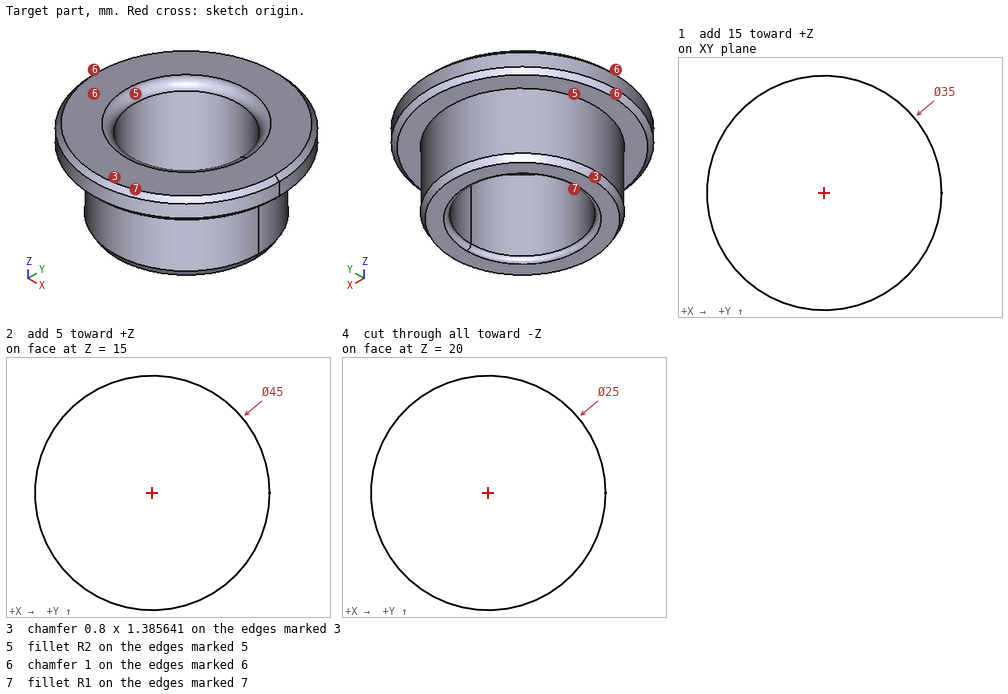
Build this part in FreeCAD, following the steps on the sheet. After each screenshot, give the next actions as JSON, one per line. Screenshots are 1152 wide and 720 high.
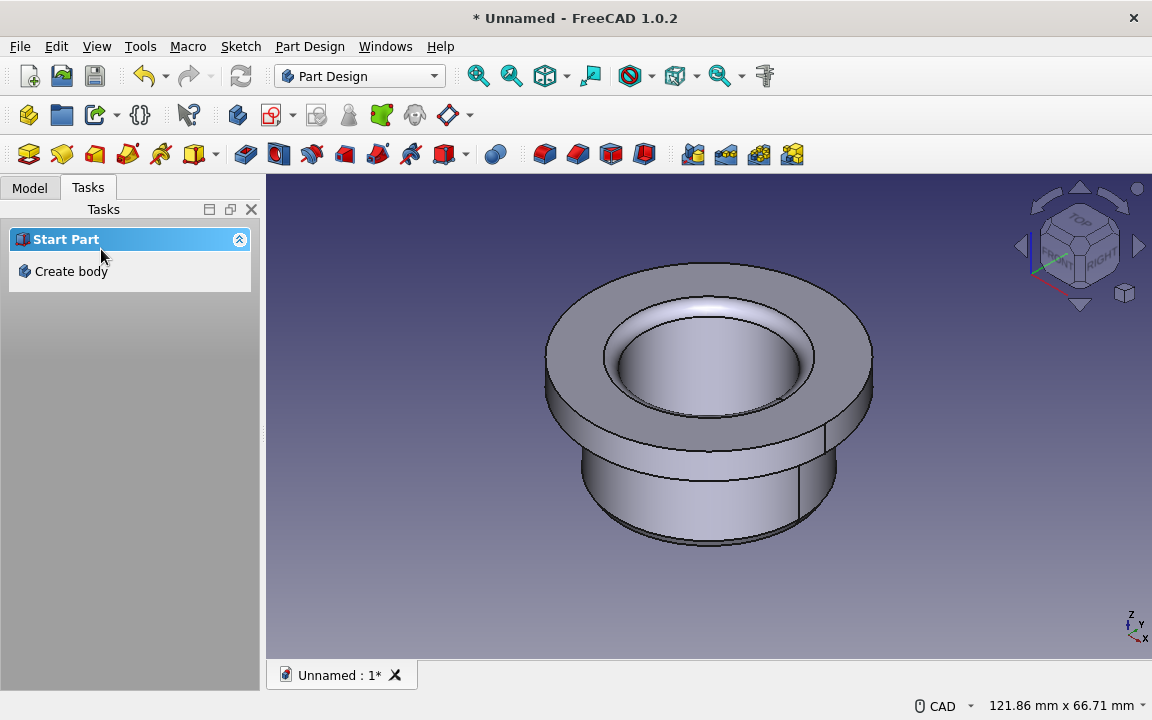
{"action": "left_click", "coordinate": [635, 470]}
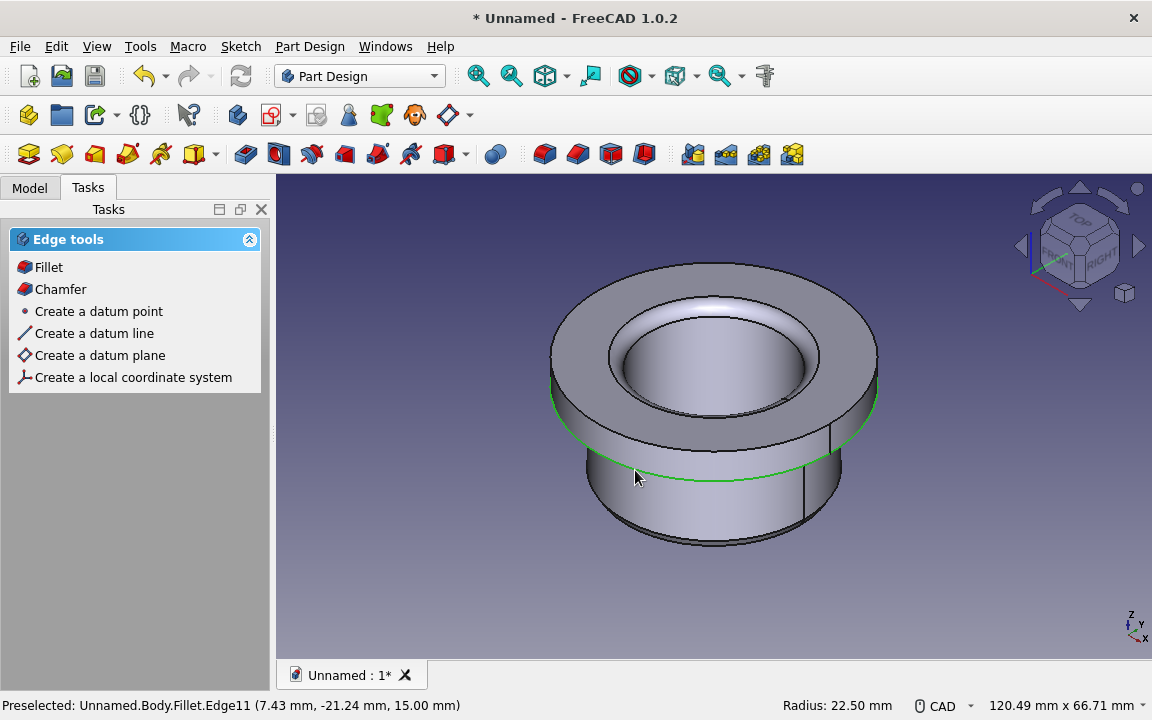
{"action": "left_click", "coordinate": [568, 399], "text": "ctrl"}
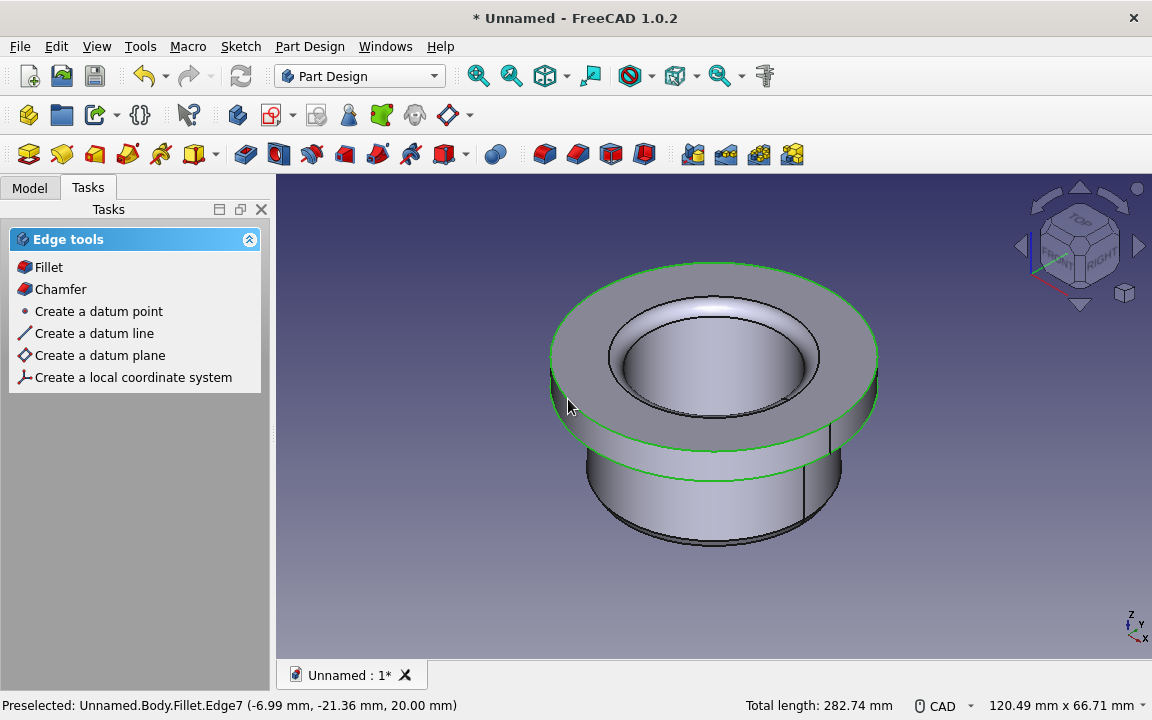
{"action": "left_click", "coordinate": [578, 154]}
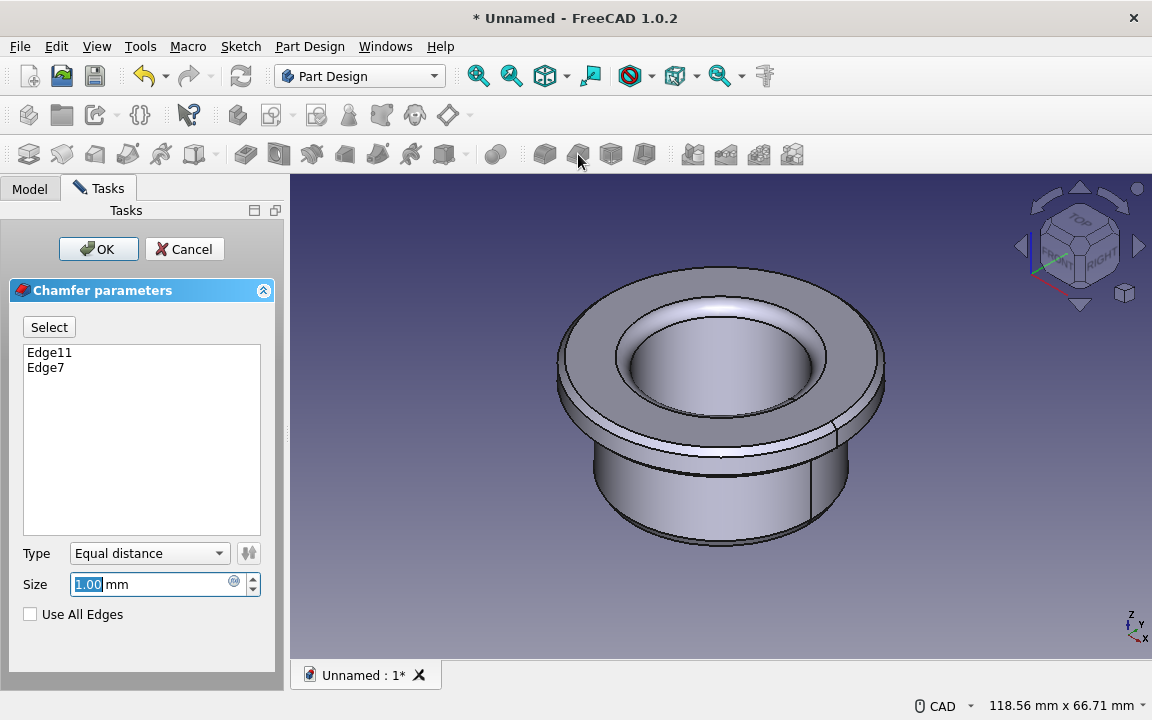
{"action": "type", "text": "1"}
{"action": "key", "text": "Tab"}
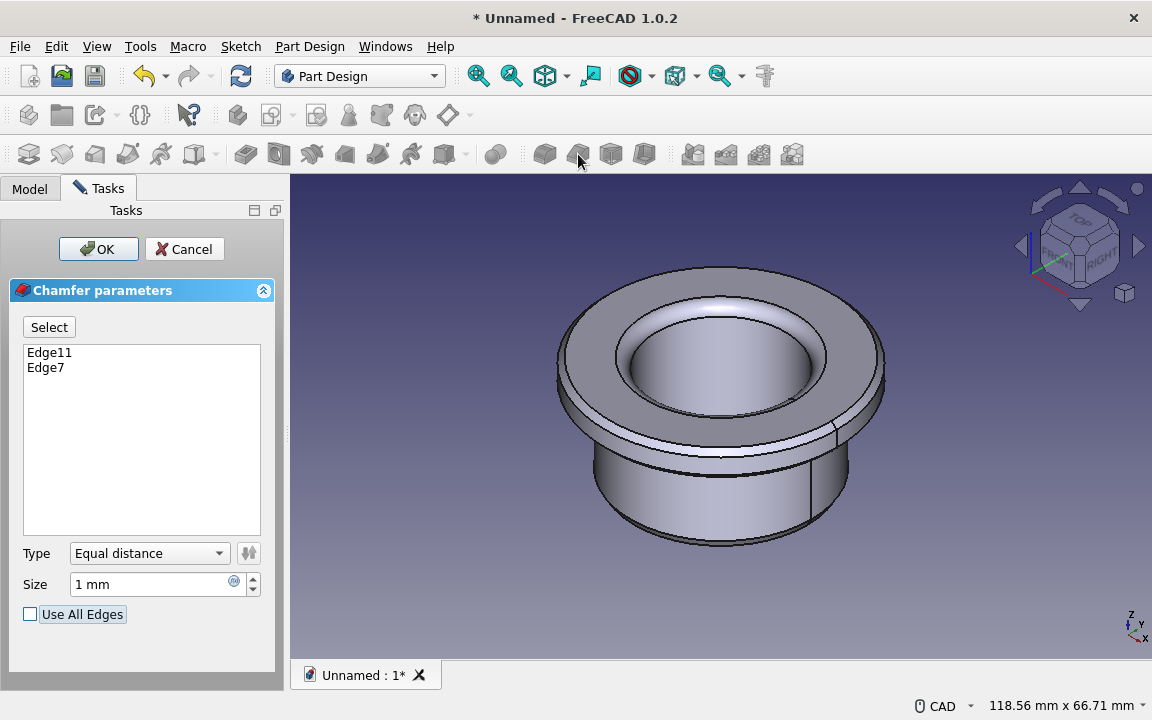
{"action": "left_click", "coordinate": [99, 249]}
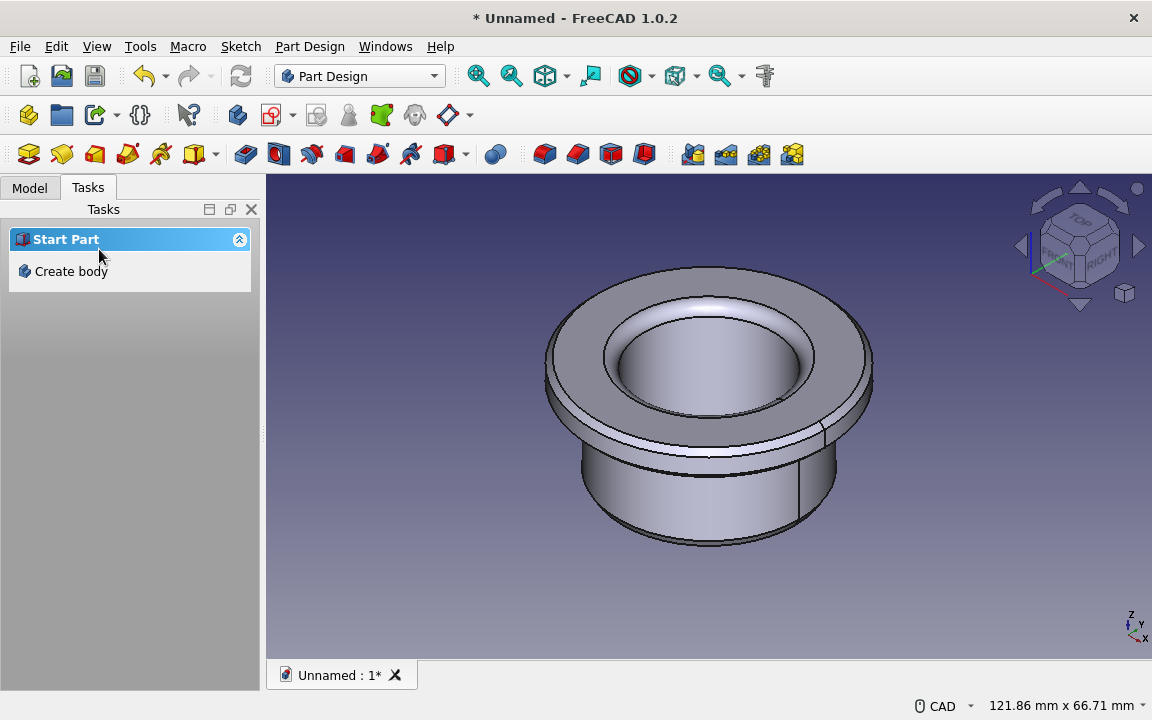
{"action": "key", "text": "2"}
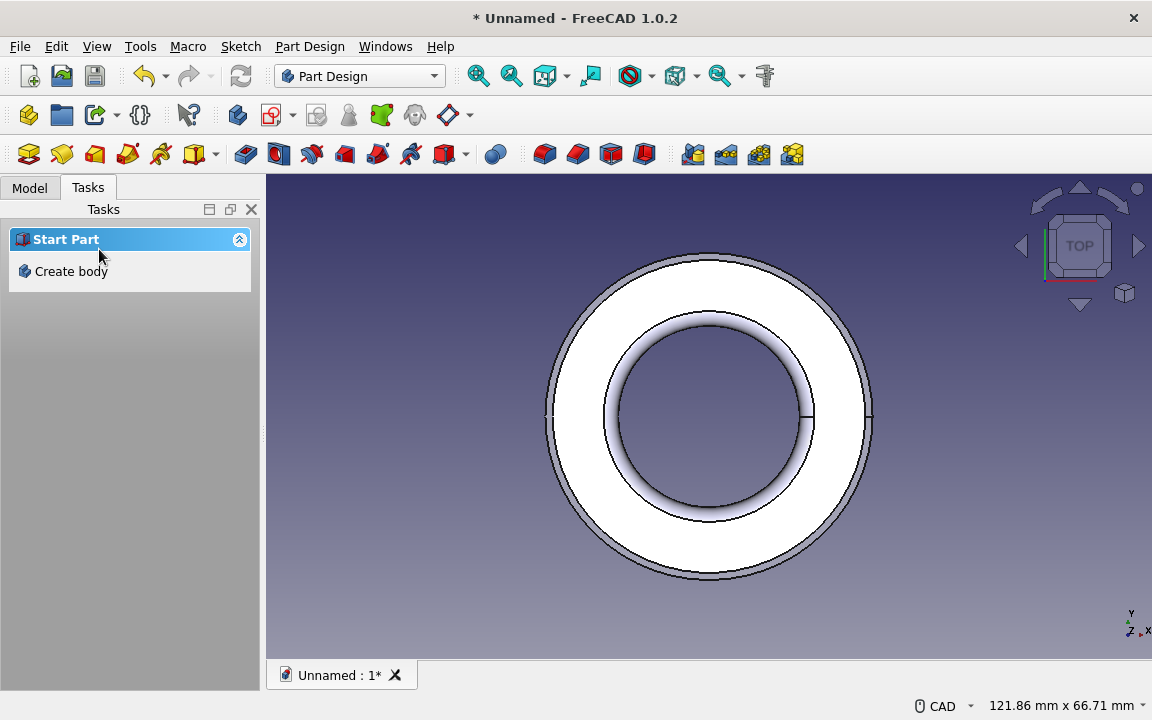
{"action": "key", "text": "0"}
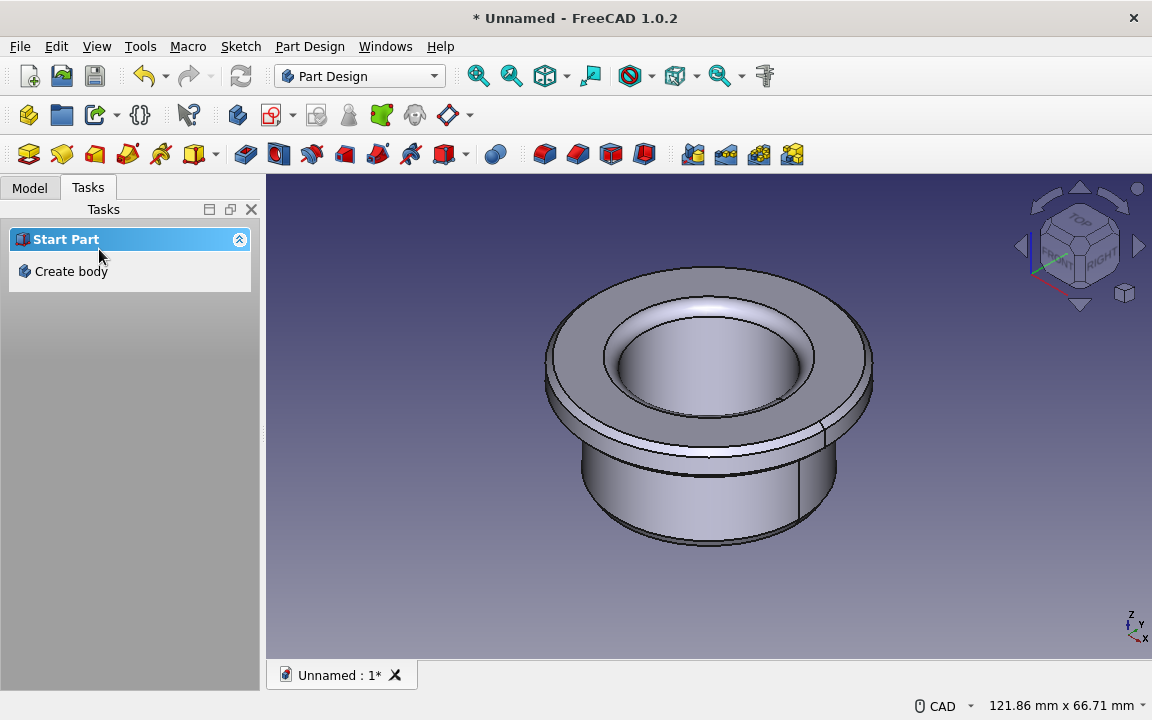
{"action": "key", "text": "1"}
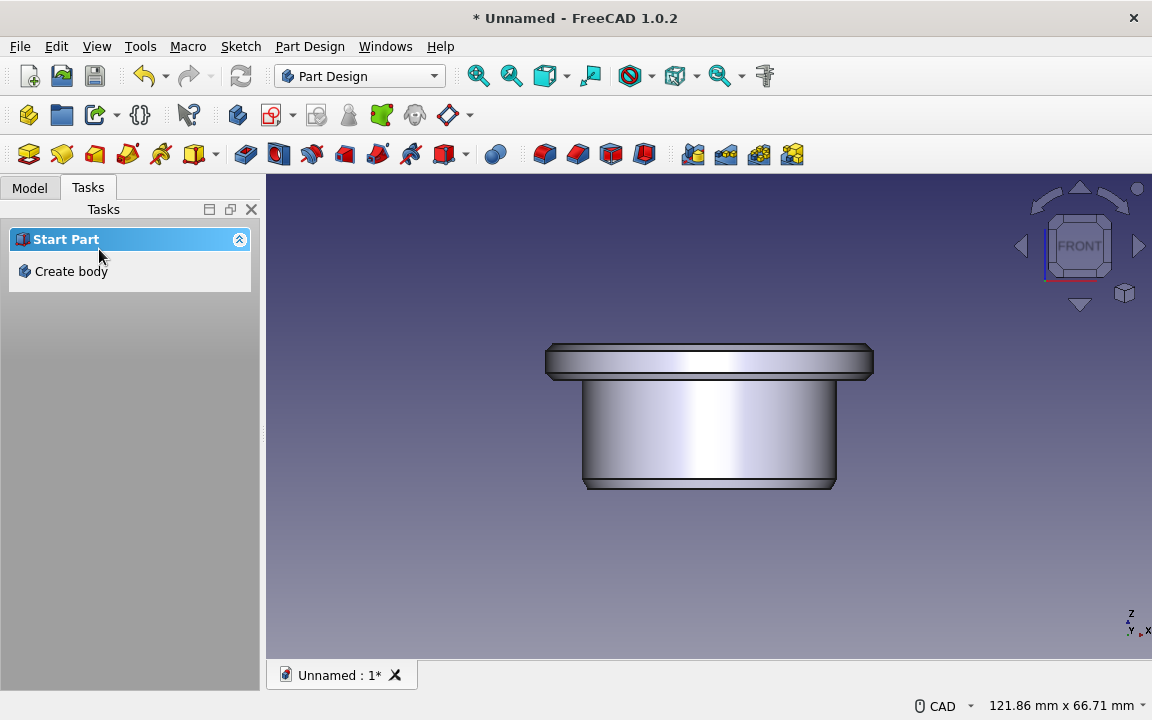
{"action": "left_click", "coordinate": [479, 76]}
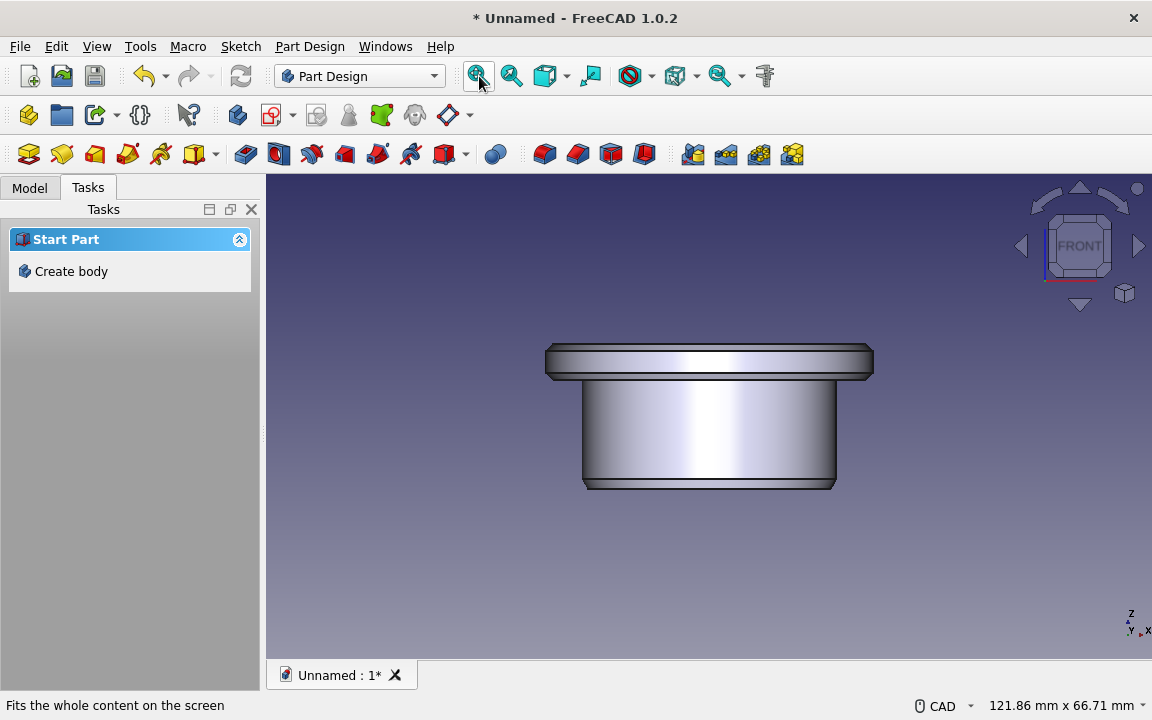
{"action": "key", "text": "3"}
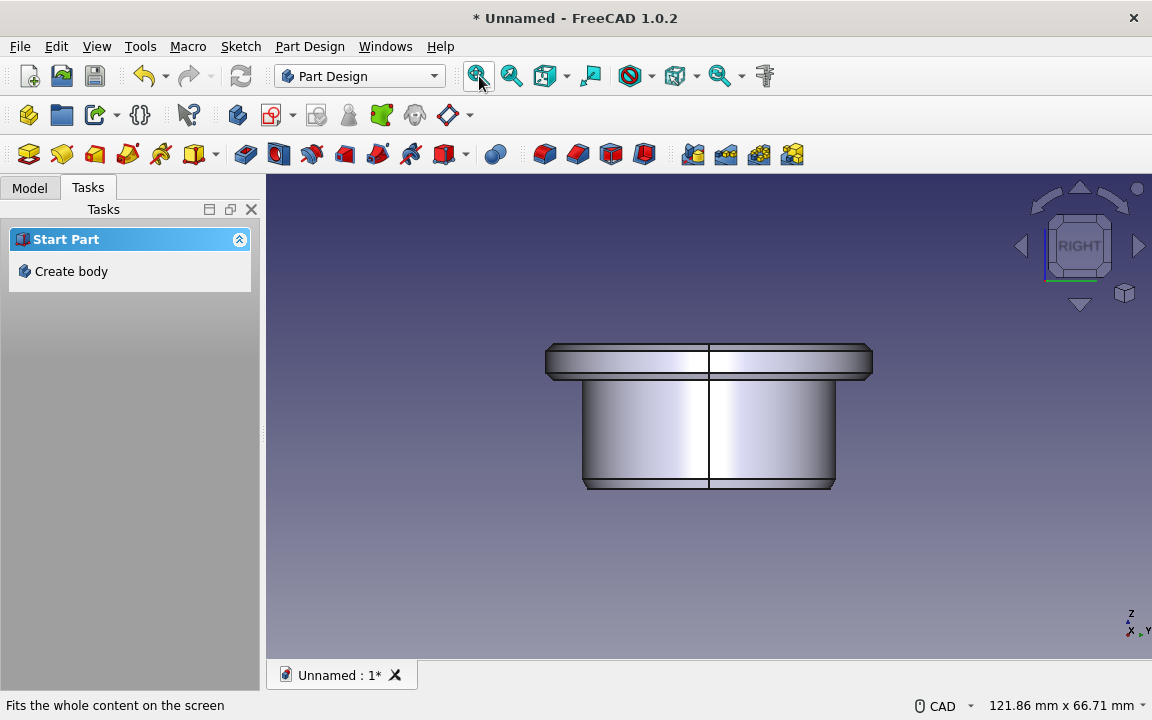
{"action": "key", "text": "v f"}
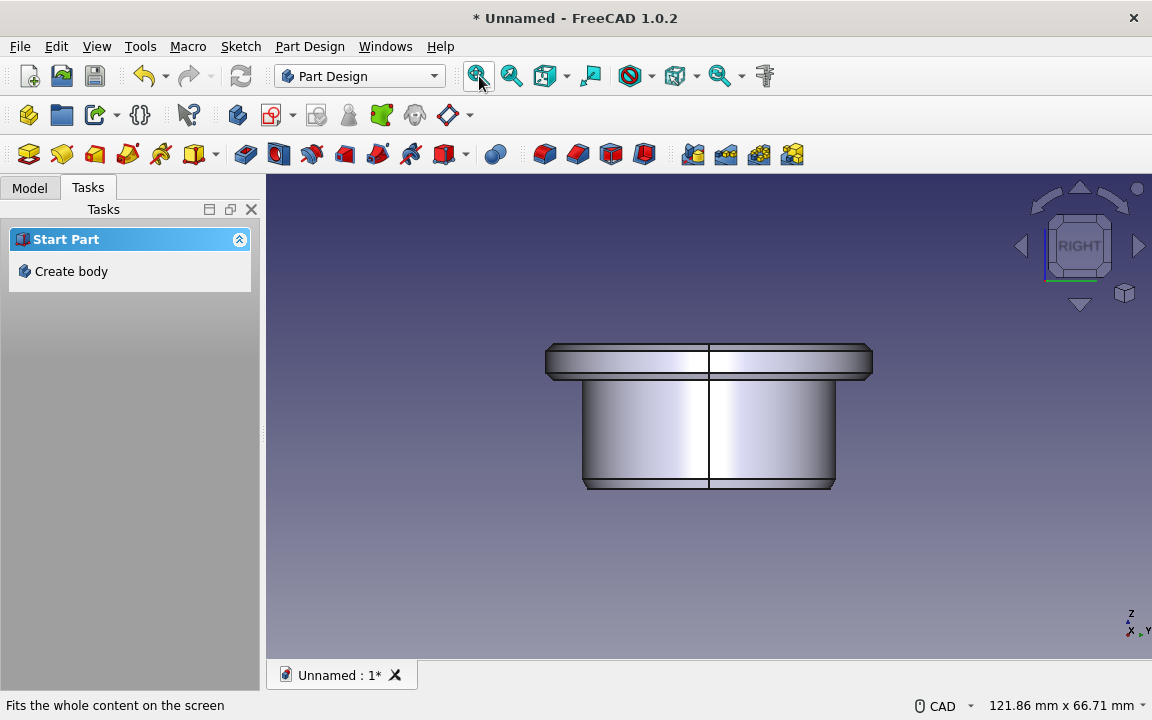
{"action": "key", "text": "5"}